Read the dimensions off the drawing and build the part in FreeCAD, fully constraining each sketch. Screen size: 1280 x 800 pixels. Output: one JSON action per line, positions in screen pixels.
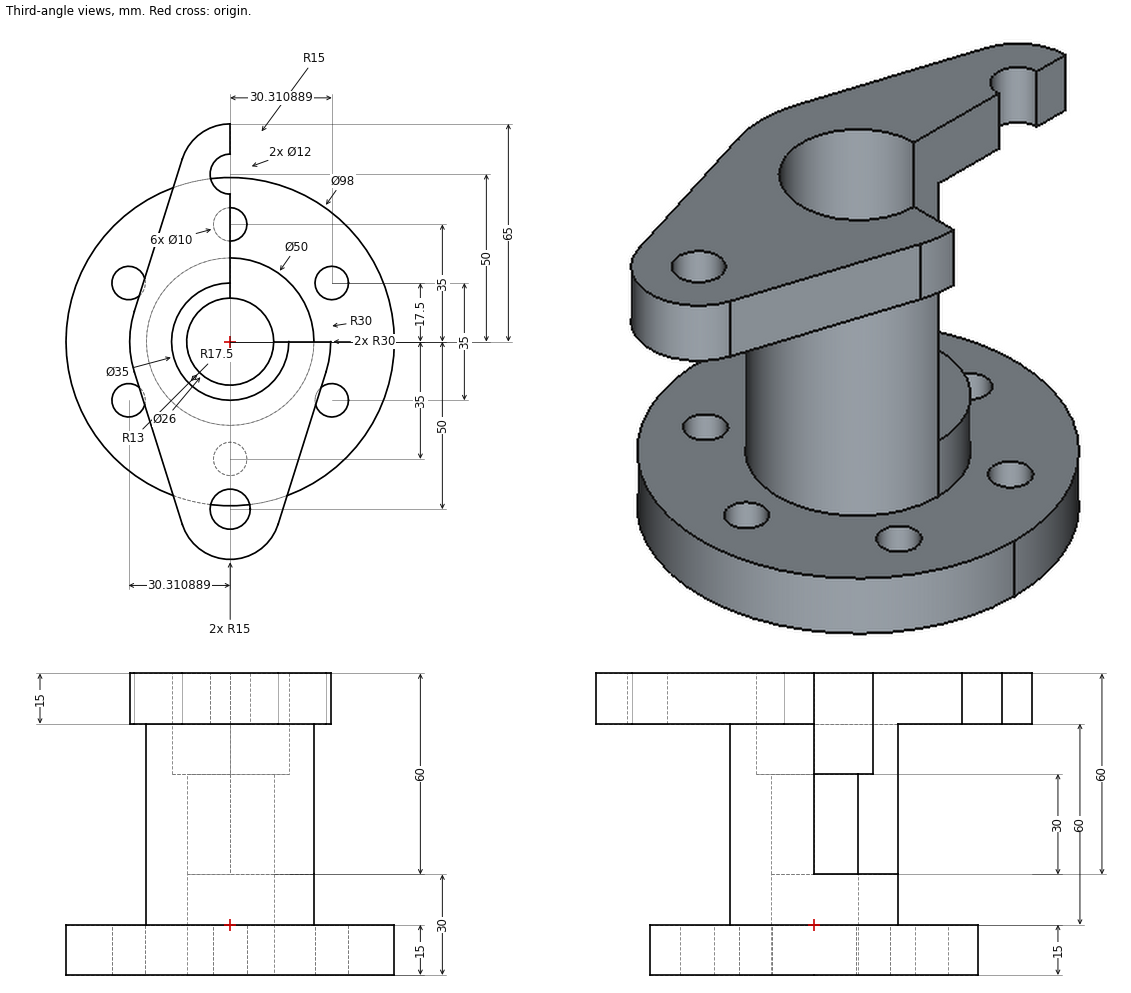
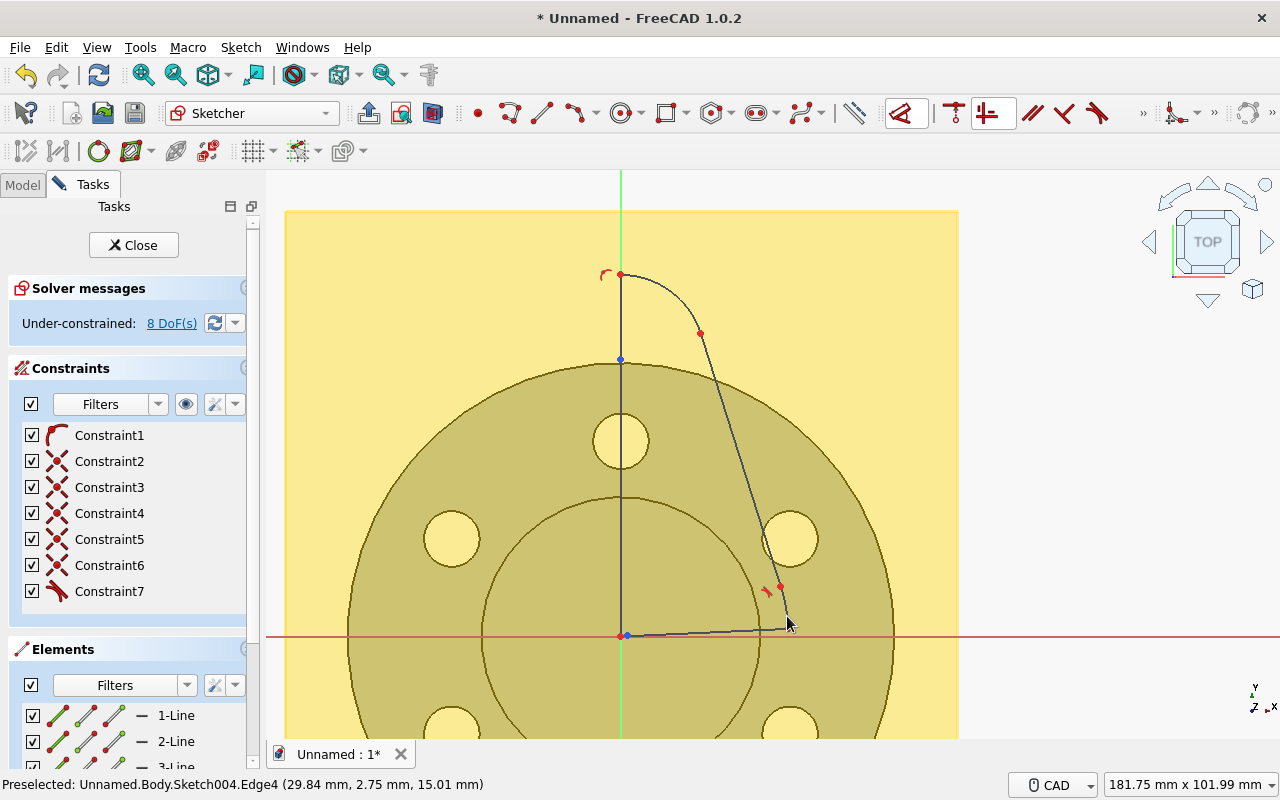
{"action": "left_click", "coordinate": [757, 511]}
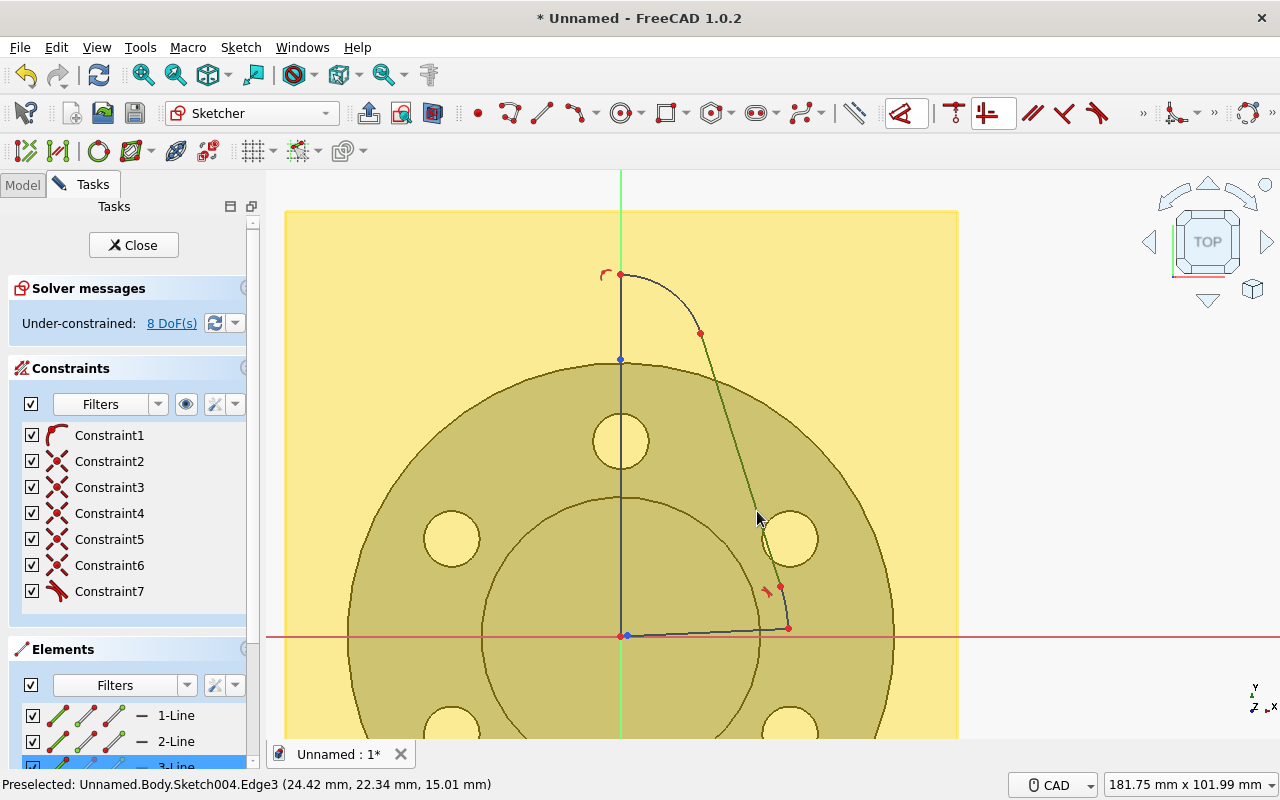
{"action": "left_click", "coordinate": [686, 306]}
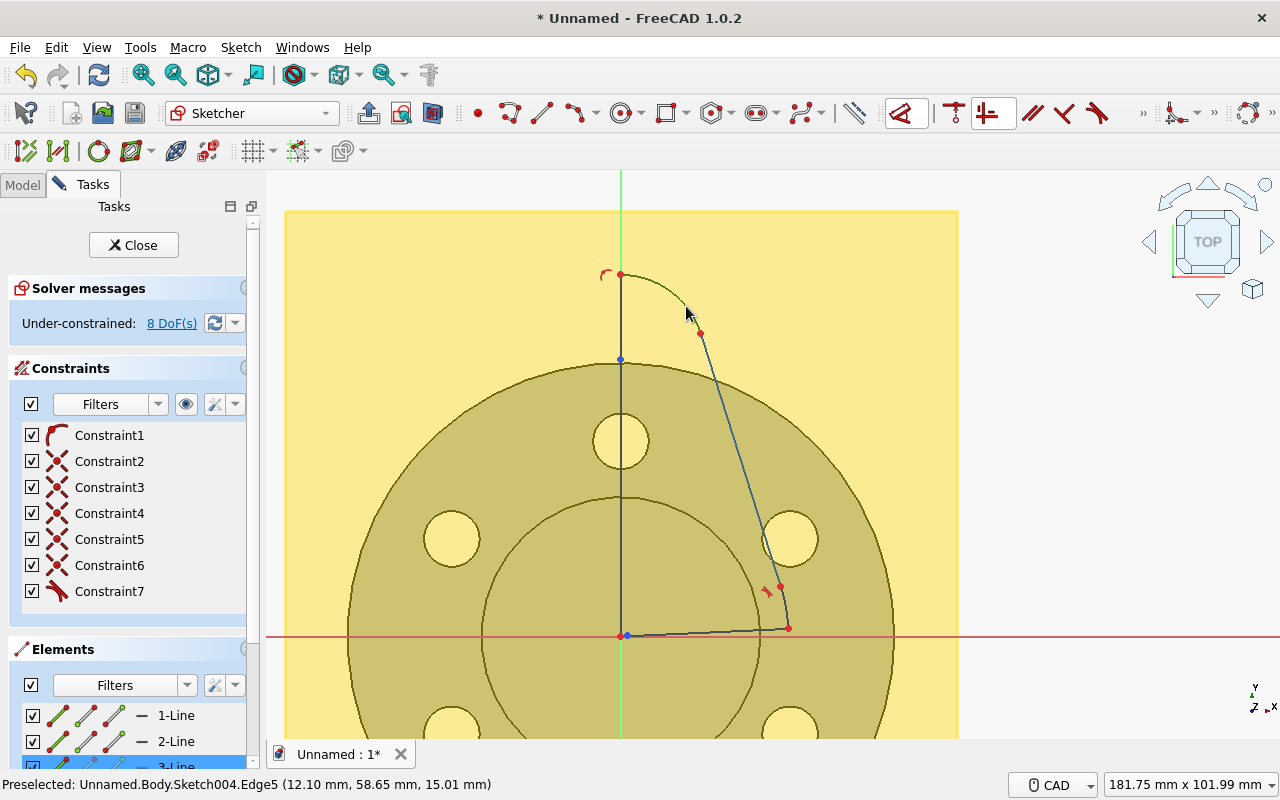
{"action": "left_click", "coordinate": [1098, 114]}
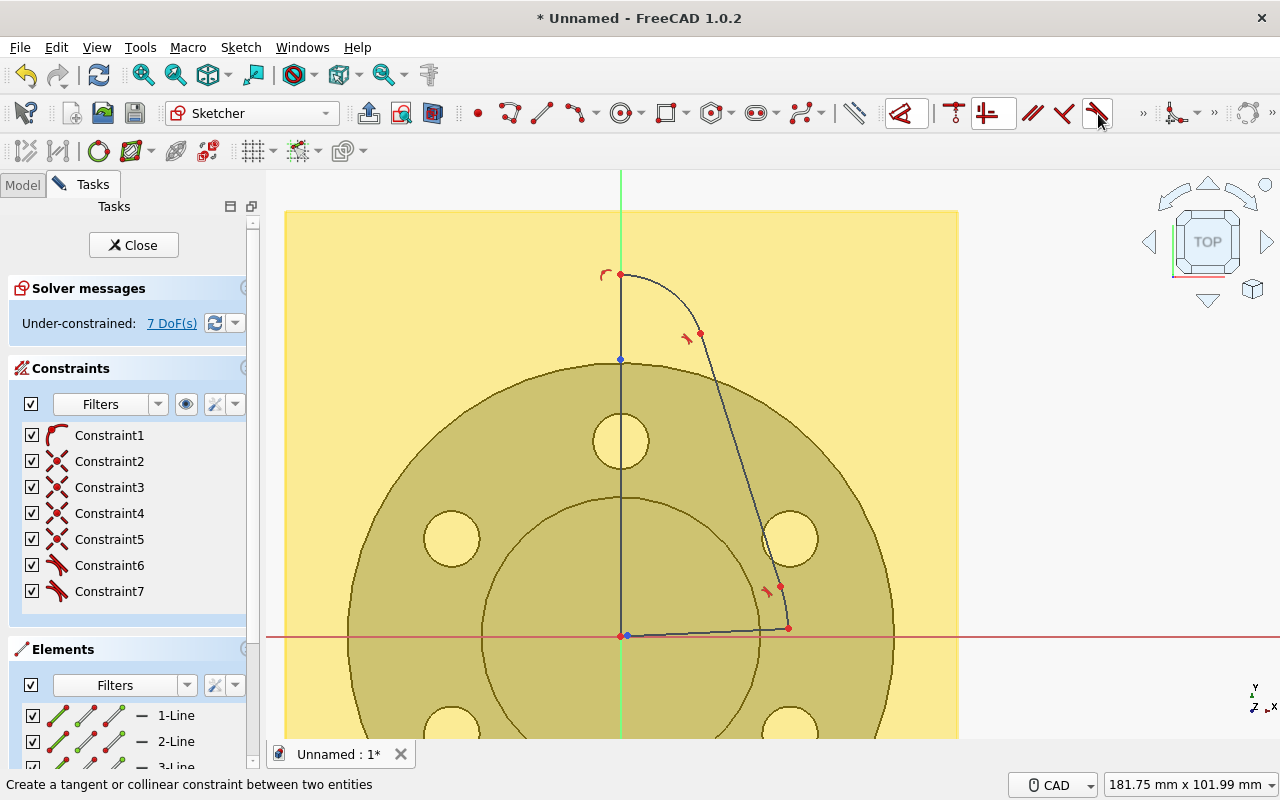
{"action": "left_click", "coordinate": [671, 634]}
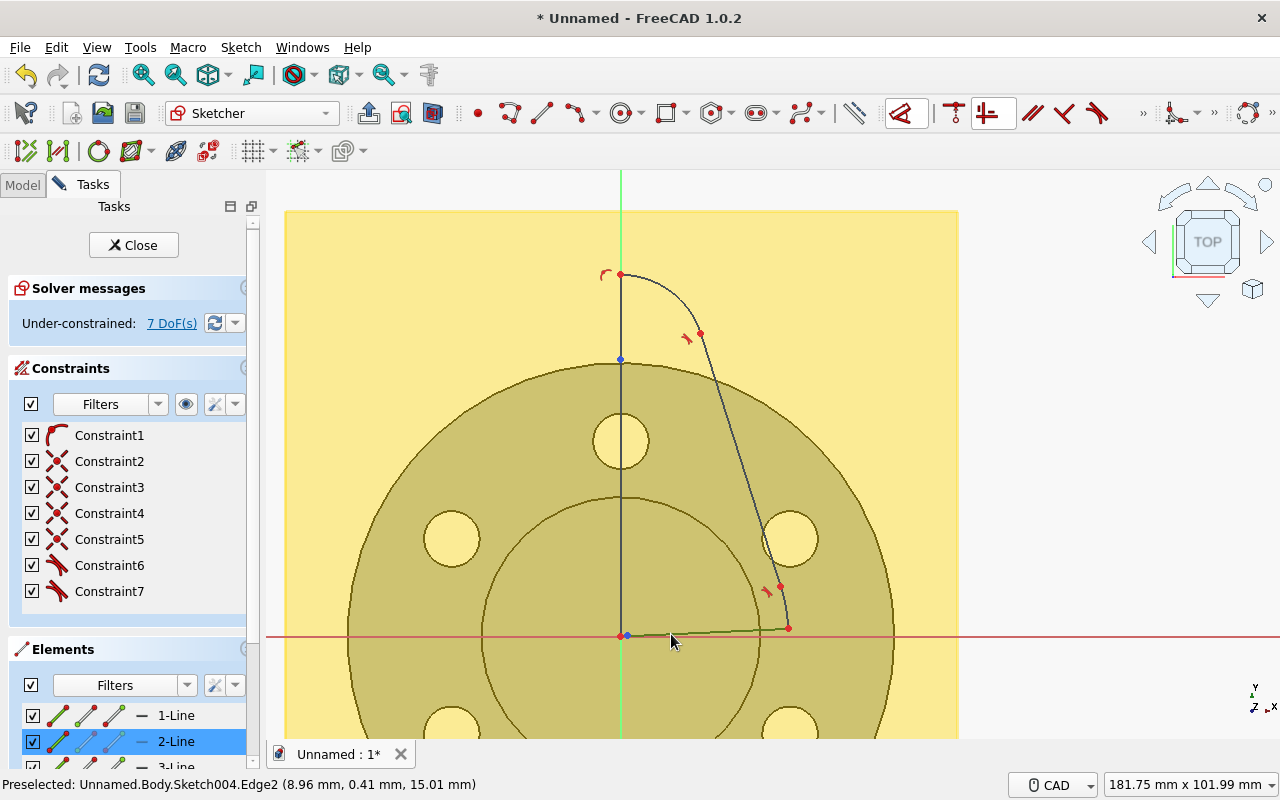
{"action": "key", "text": "h"}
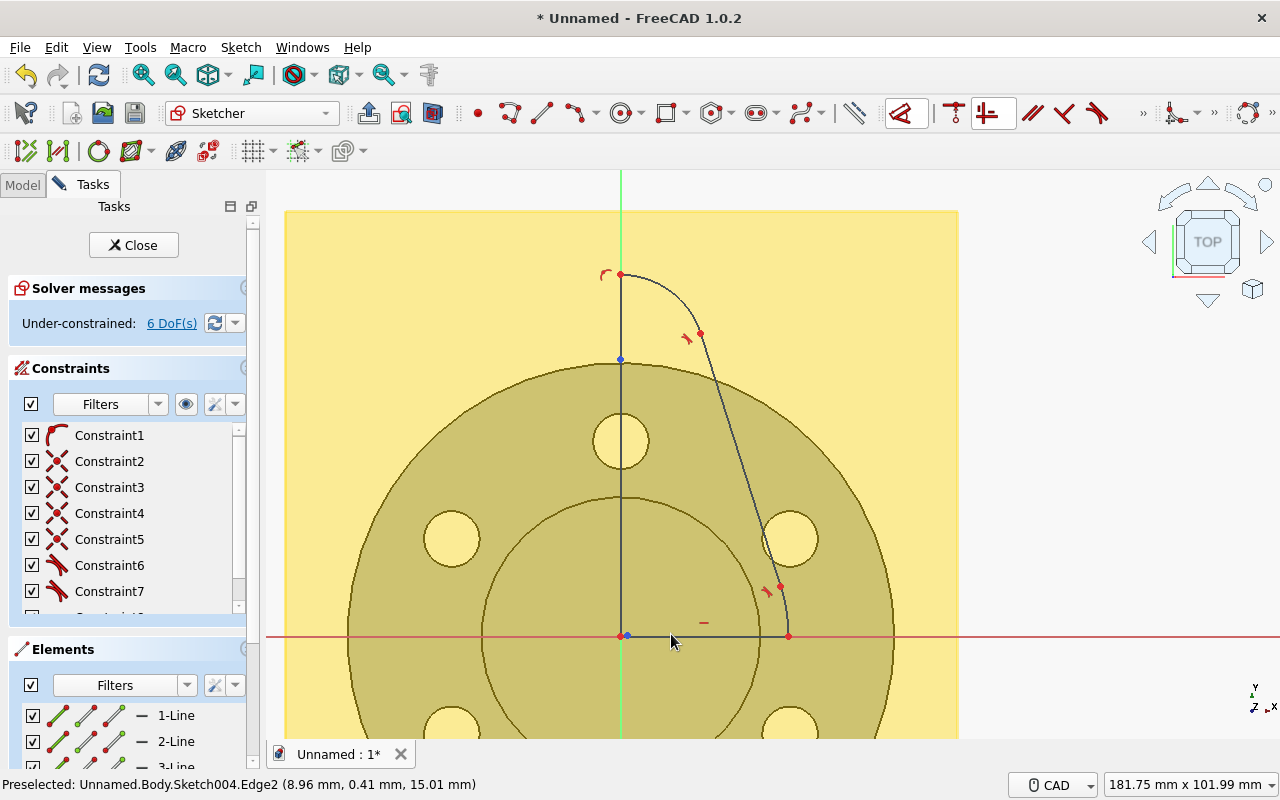
{"action": "scroll", "coordinate": [624, 636], "scroll_direction": "up", "scroll_amount": 13}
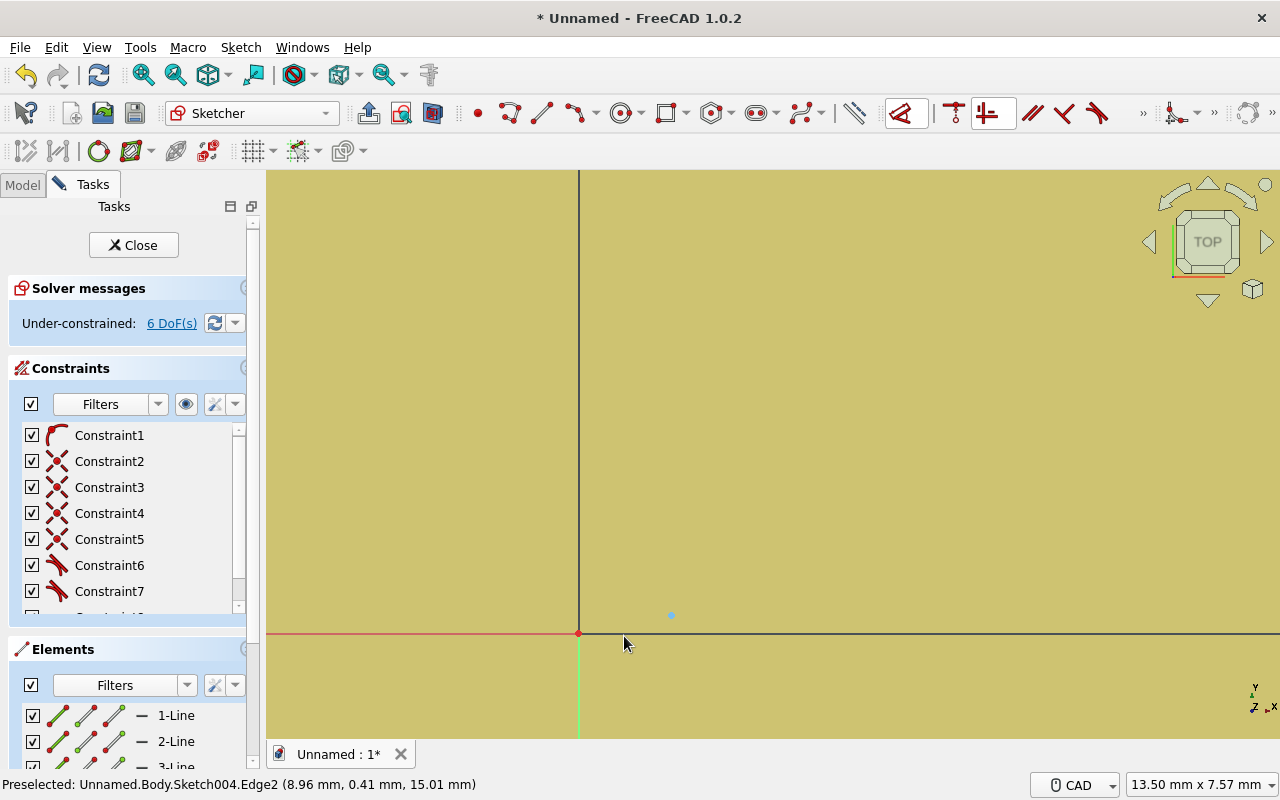
{"action": "left_click_drag", "start_coordinate": [569, 606], "coordinate": [682, 644]}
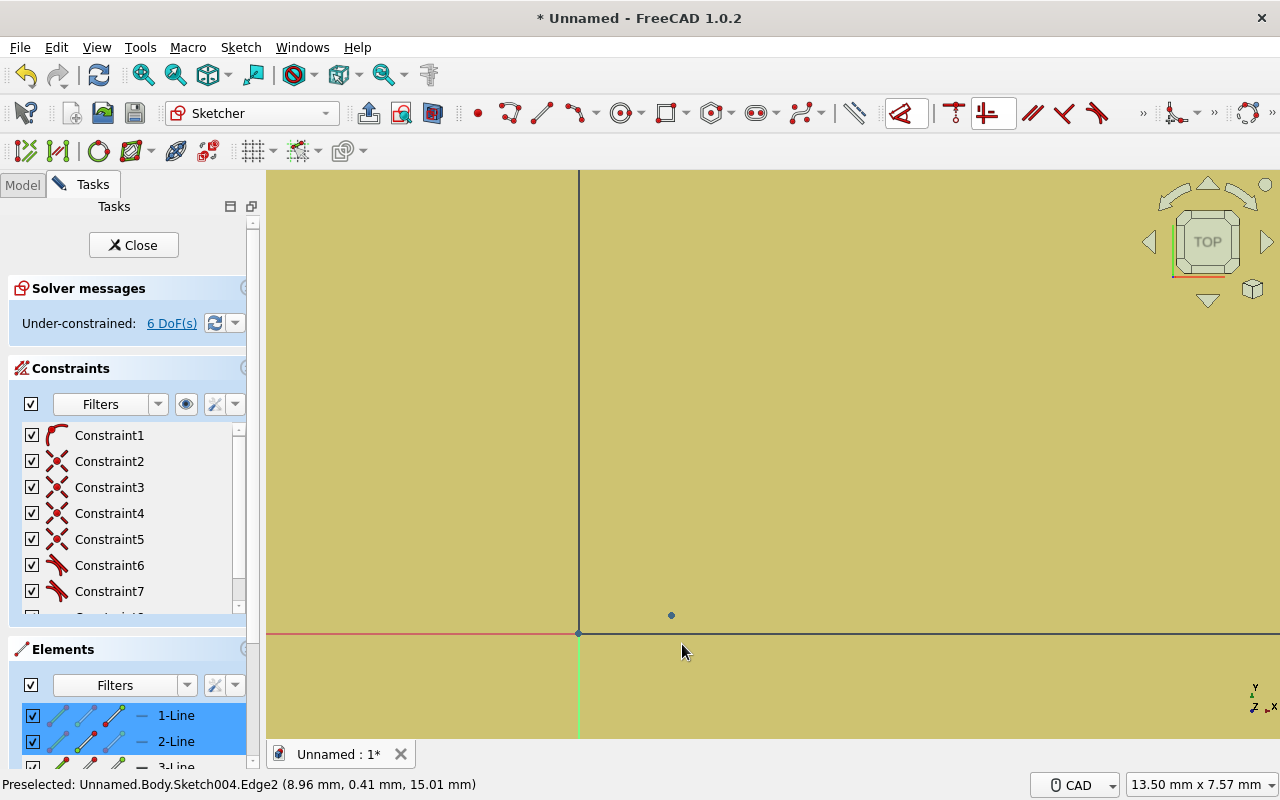
{"action": "key", "text": "c"}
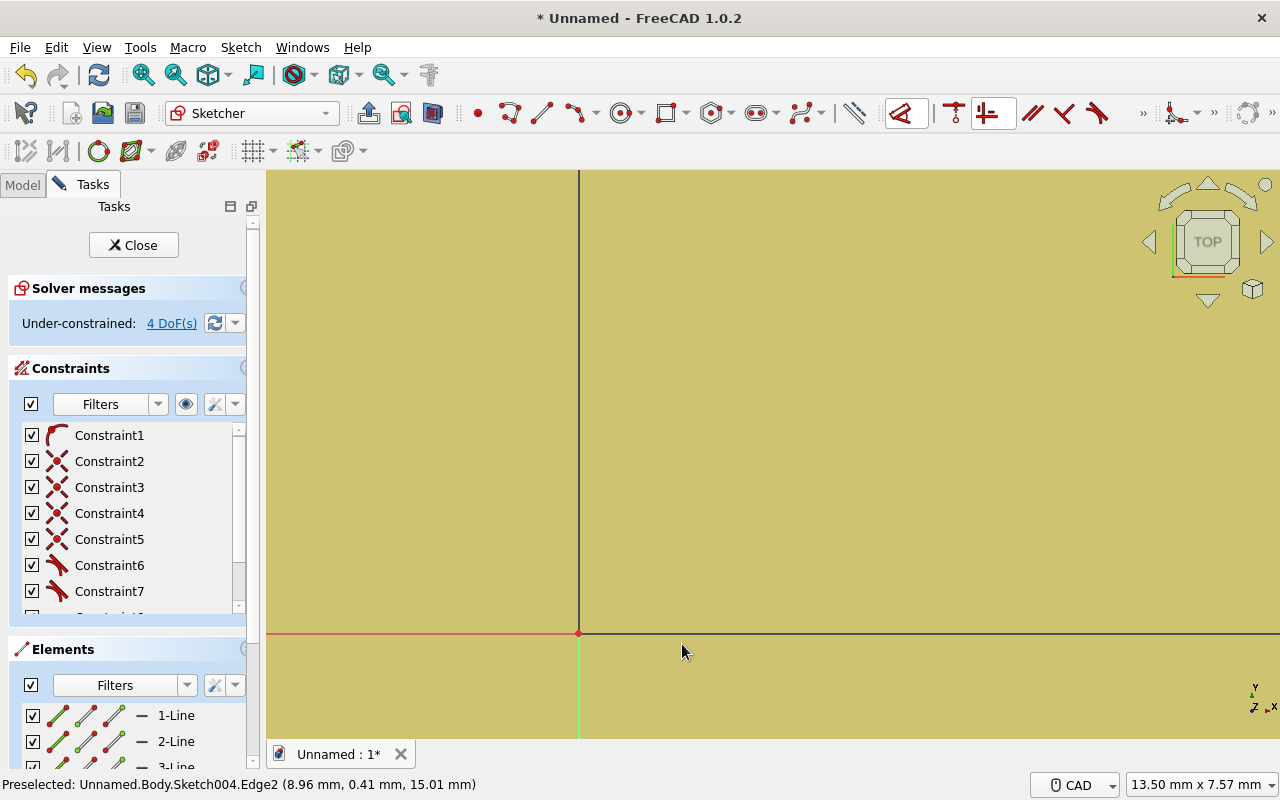
{"action": "scroll", "coordinate": [624, 636], "scroll_direction": "down", "scroll_amount": 13}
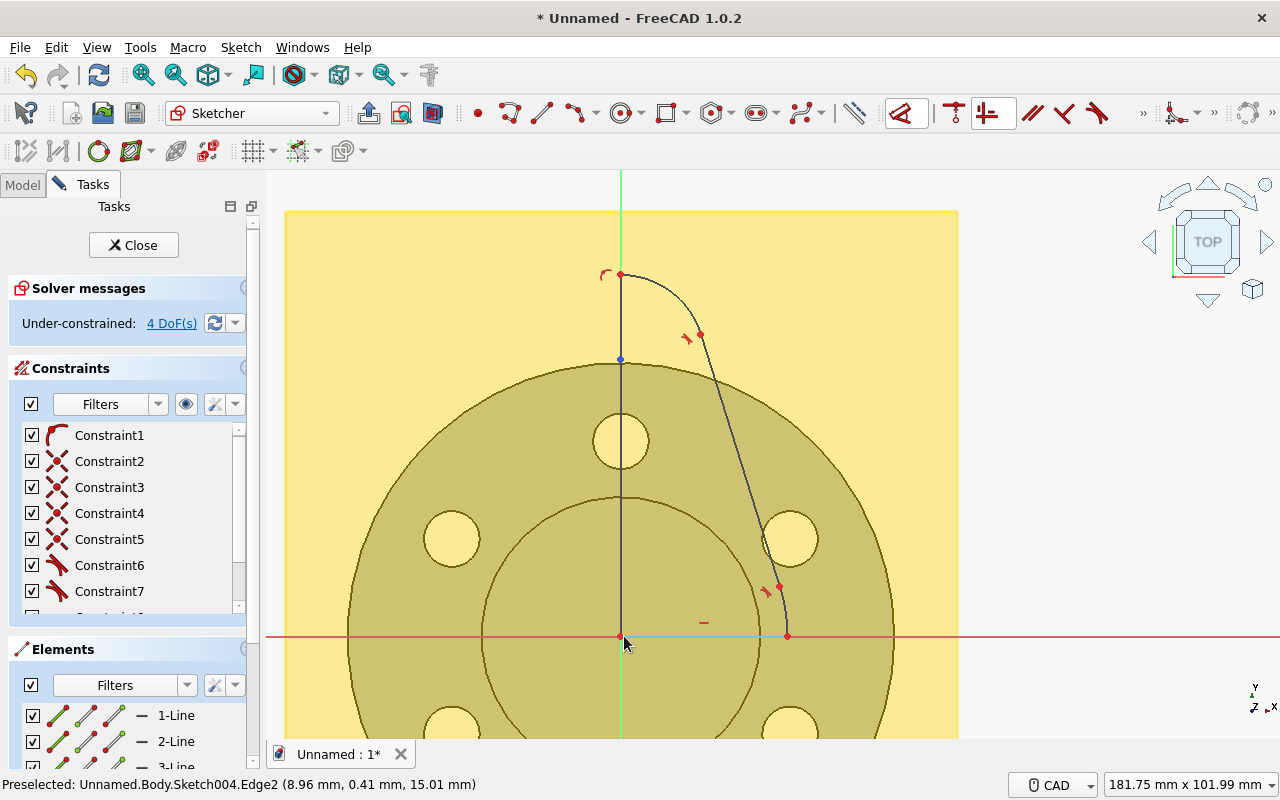
{"action": "left_click", "coordinate": [620, 359]}